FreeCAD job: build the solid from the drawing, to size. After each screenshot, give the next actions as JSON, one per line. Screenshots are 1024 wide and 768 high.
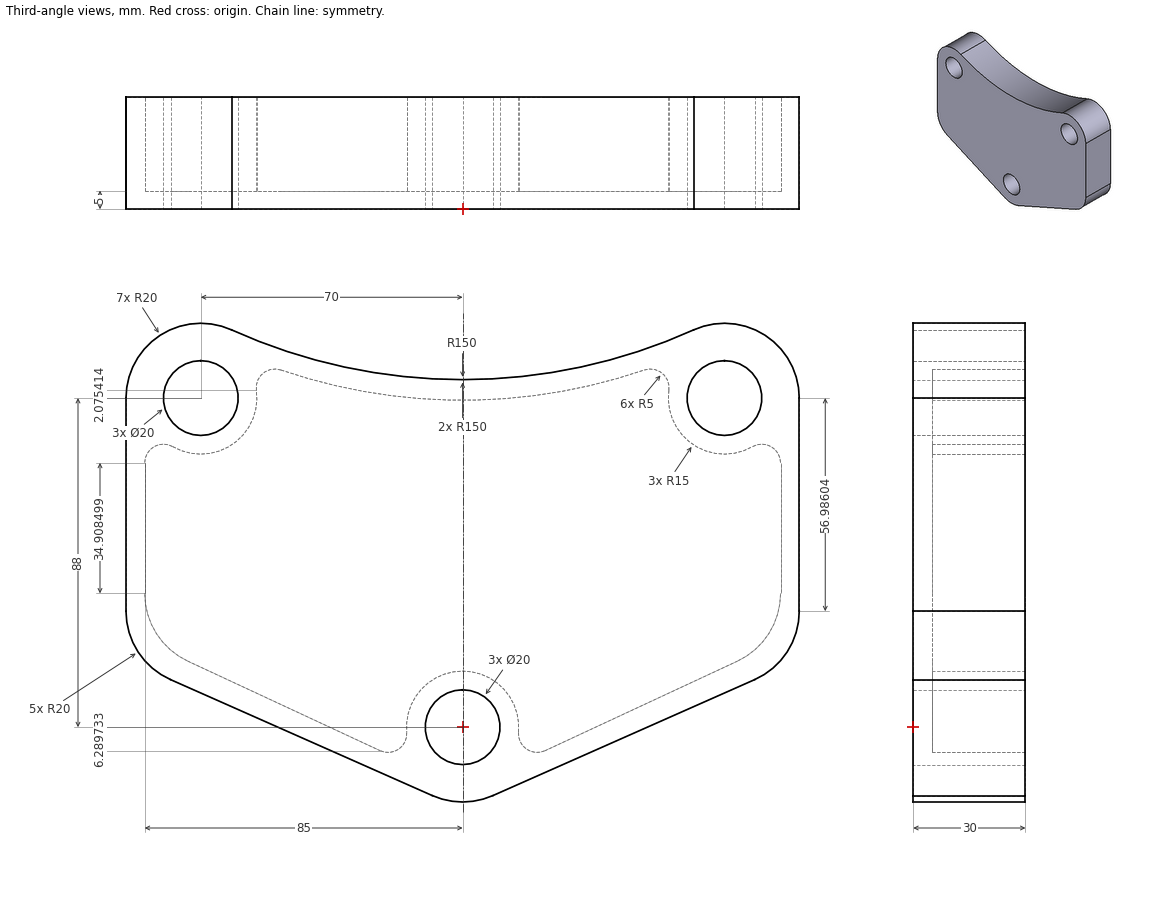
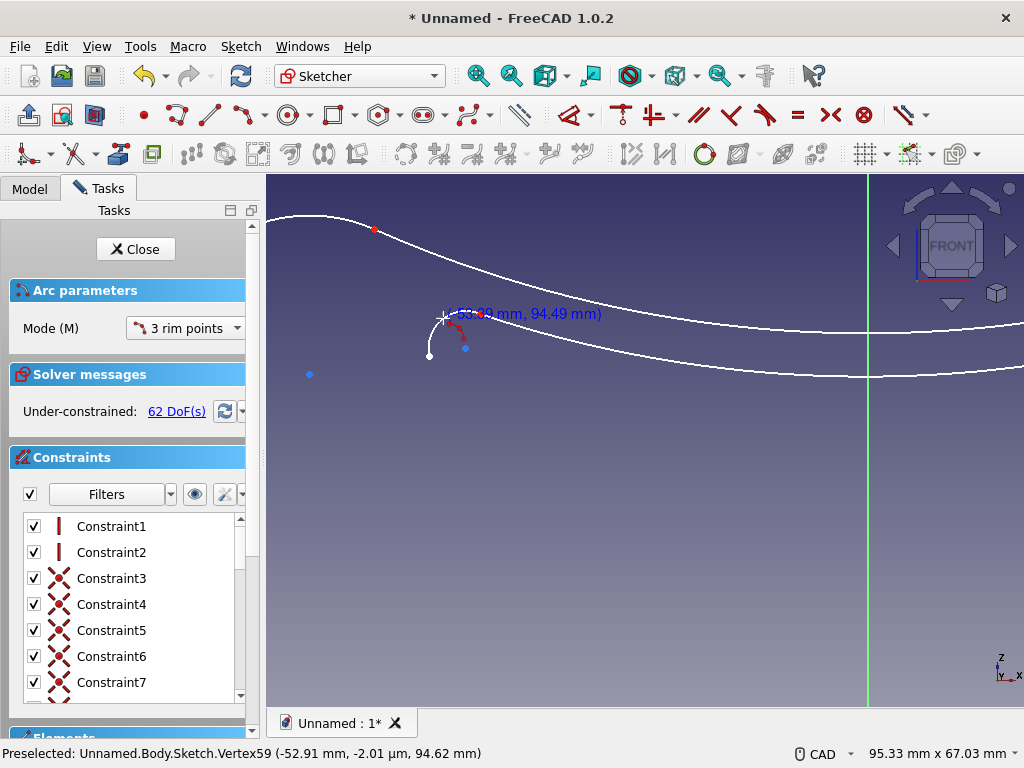
{"action": "left_click", "coordinate": [429, 357]}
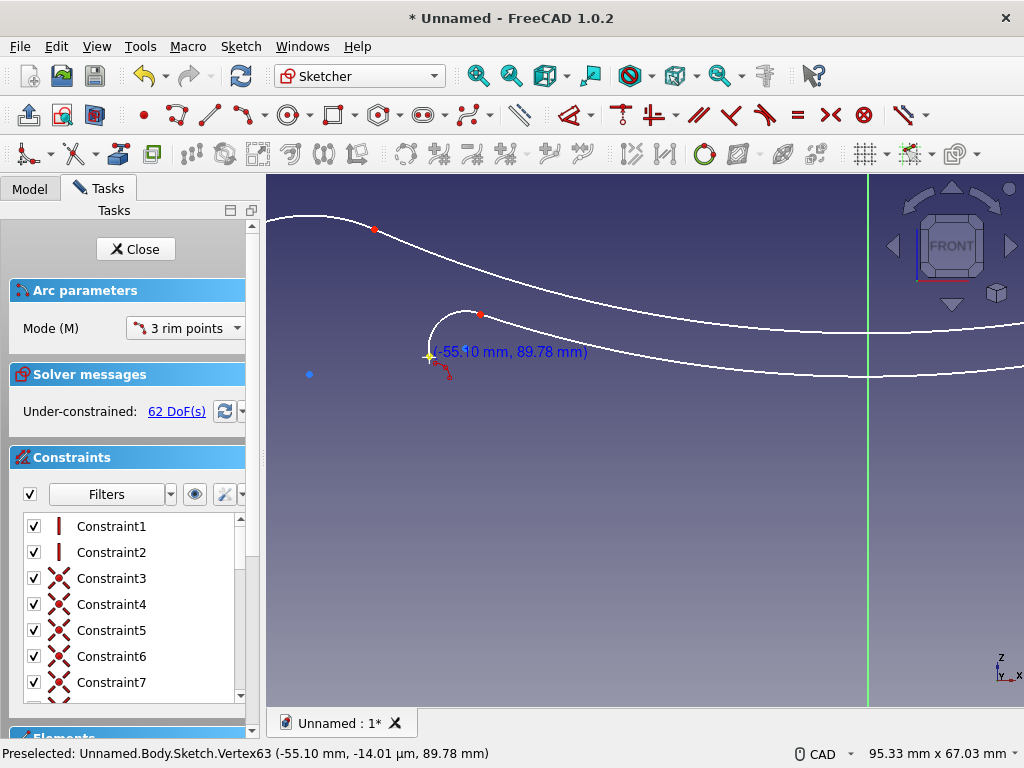
{"action": "scroll", "coordinate": [451, 317], "scroll_direction": "down", "scroll_amount": 6}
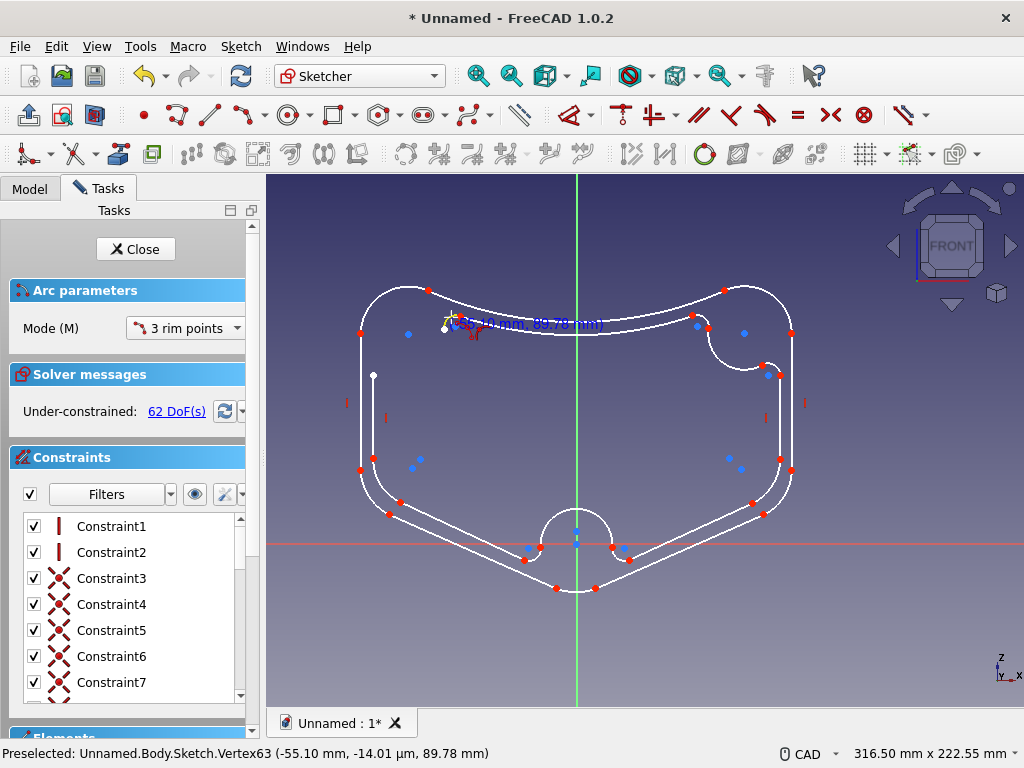
{"action": "left_click", "coordinate": [391, 364]}
{"action": "left_click", "coordinate": [429, 363]}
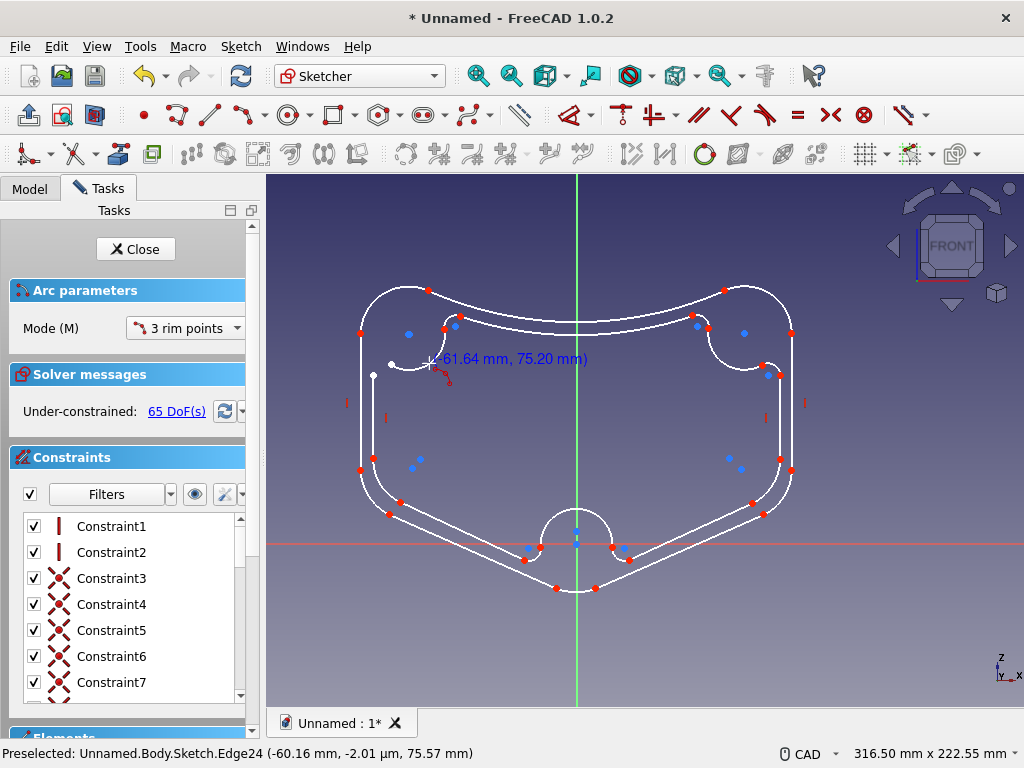
{"action": "left_click", "coordinate": [391, 365]}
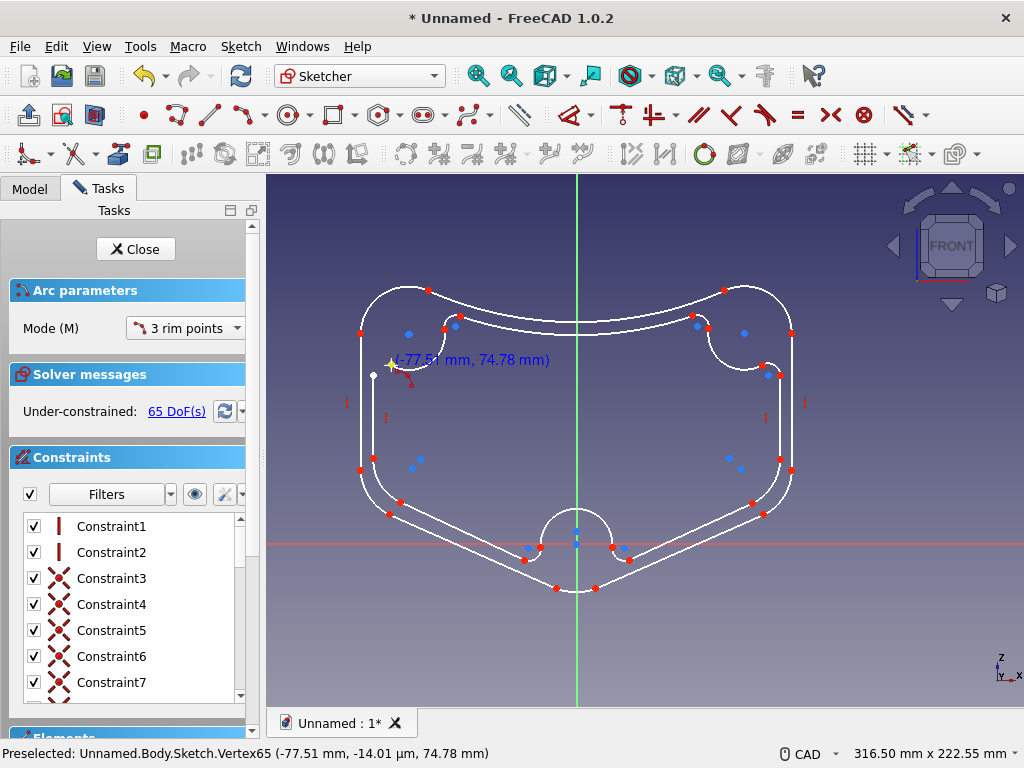
{"action": "scroll", "coordinate": [373, 375], "scroll_direction": "up", "scroll_amount": 2}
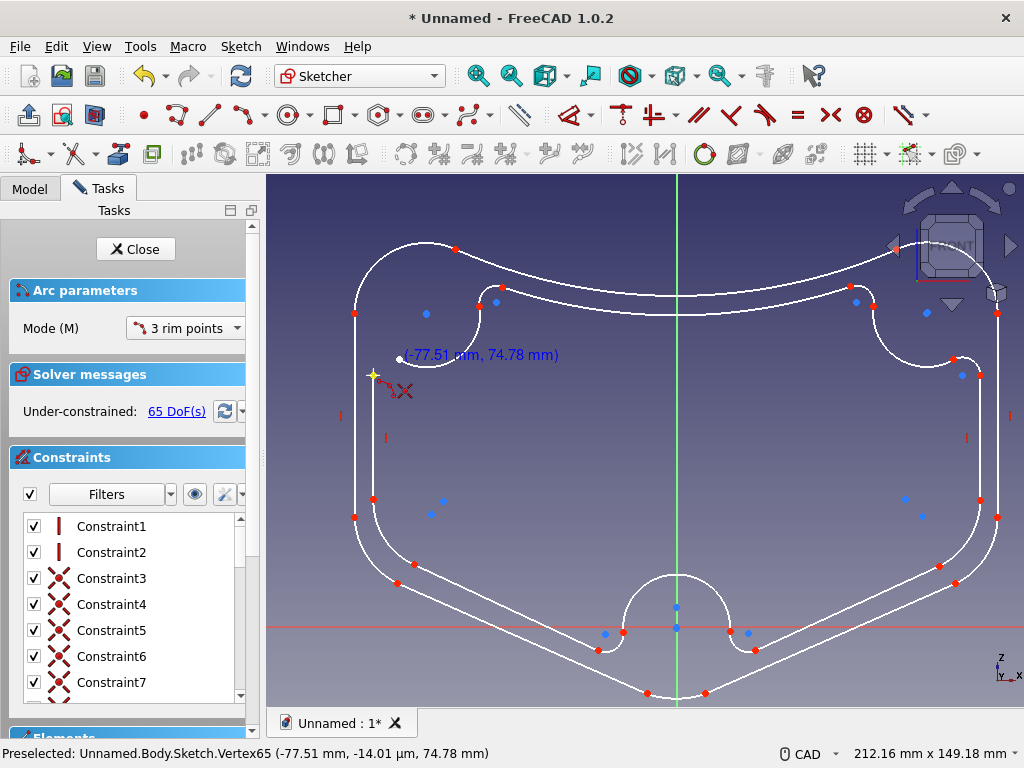
{"action": "left_click", "coordinate": [373, 376]}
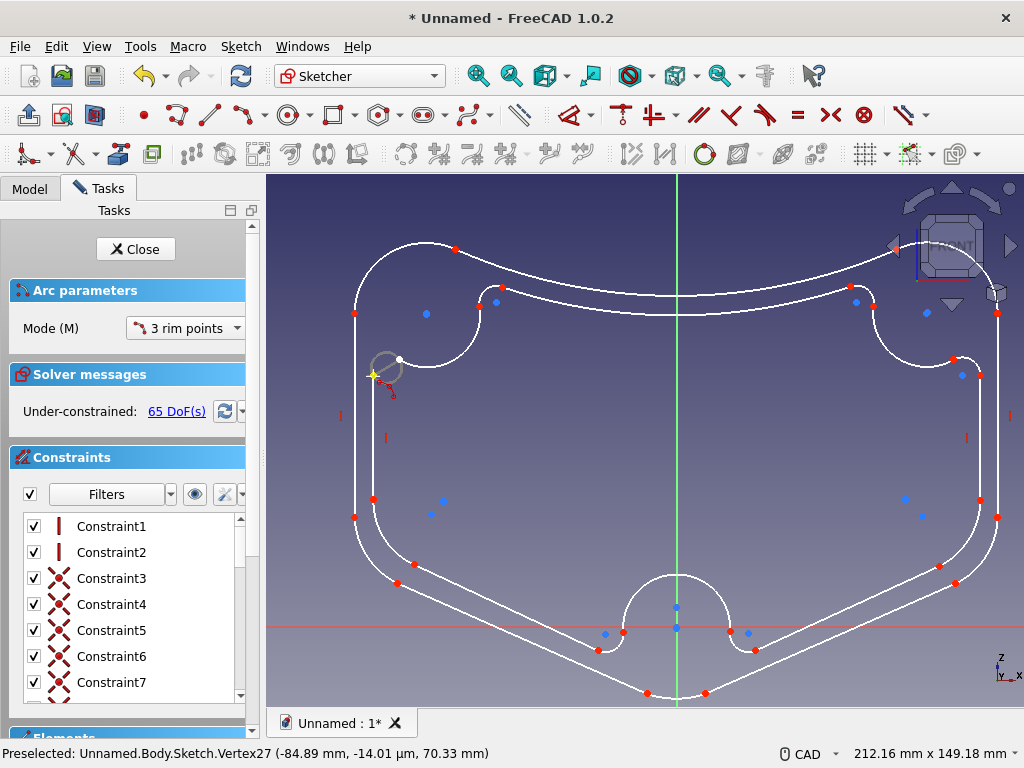
{"action": "scroll", "coordinate": [382, 359], "scroll_direction": "up", "scroll_amount": 3}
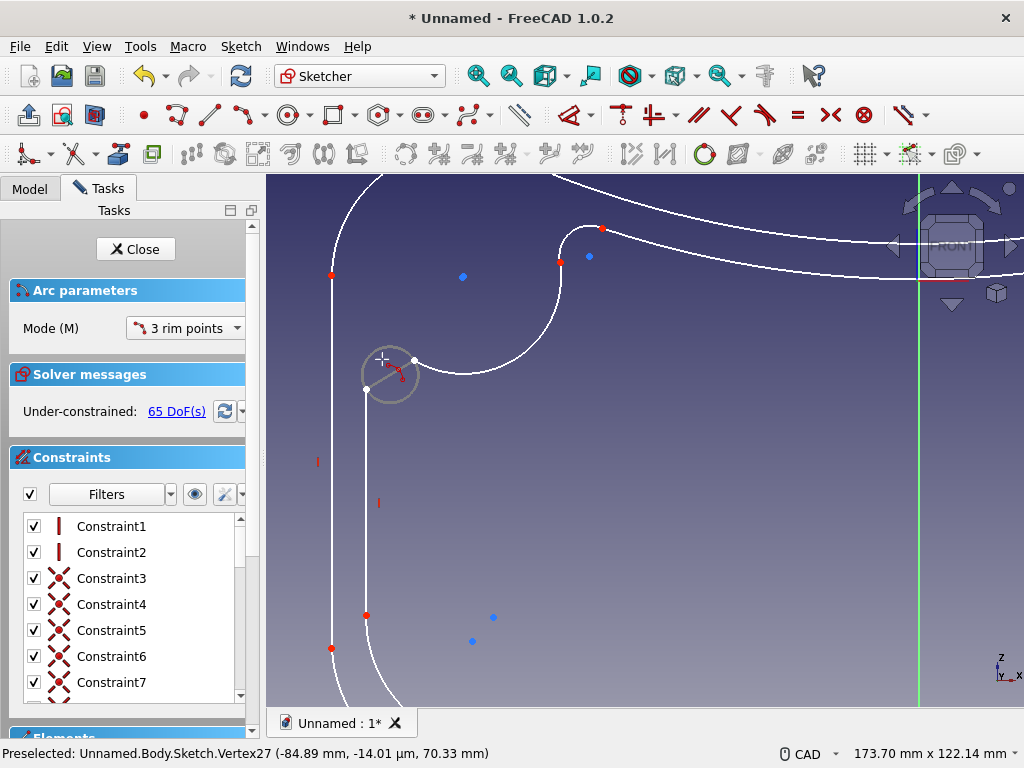
{"action": "left_click", "coordinate": [382, 359]}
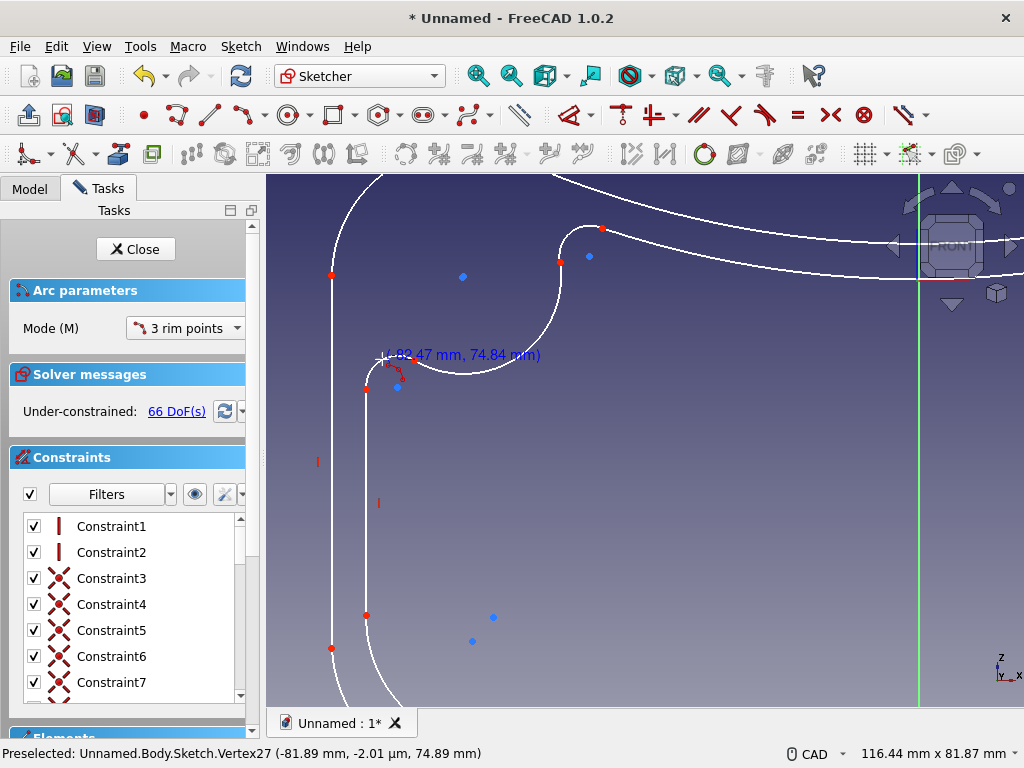
{"action": "left_click", "coordinate": [288, 116]}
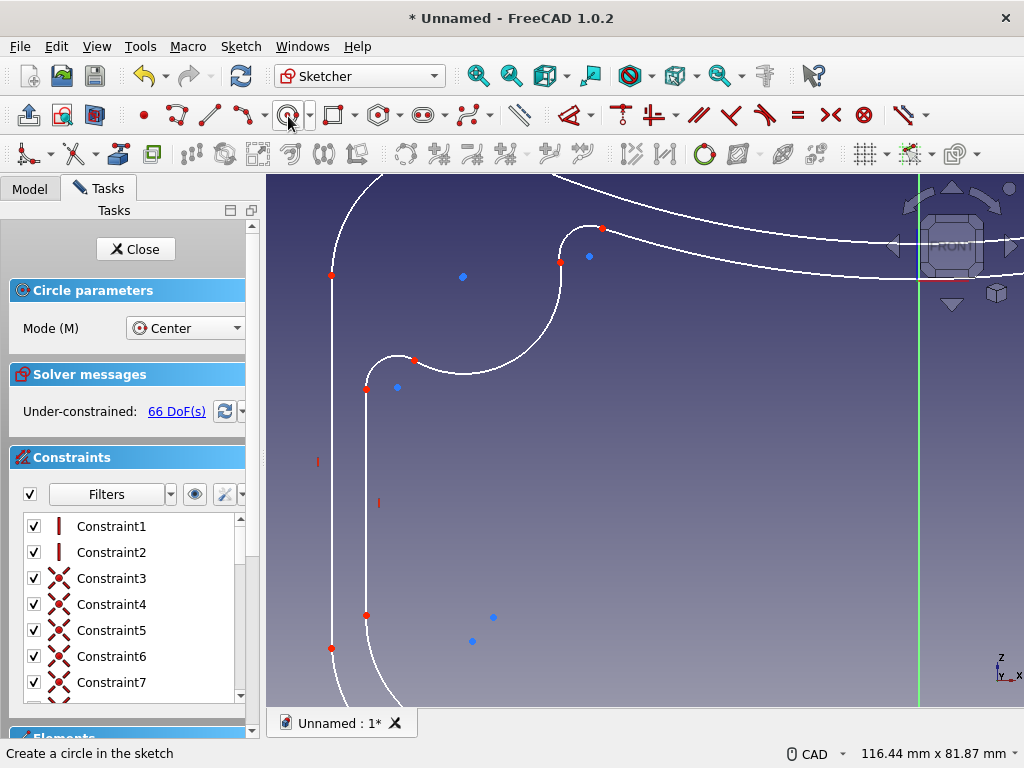
{"action": "left_click", "coordinate": [463, 274]}
{"action": "left_click", "coordinate": [509, 228]}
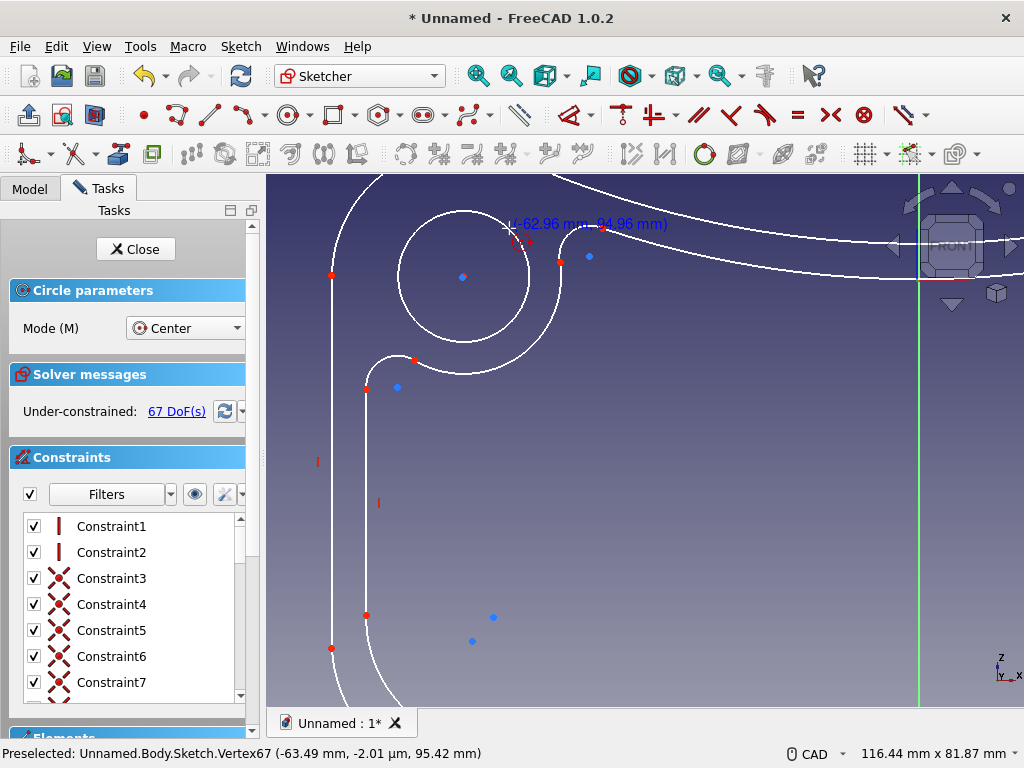
{"action": "scroll", "coordinate": [377, 367], "scroll_direction": "down", "scroll_amount": 5}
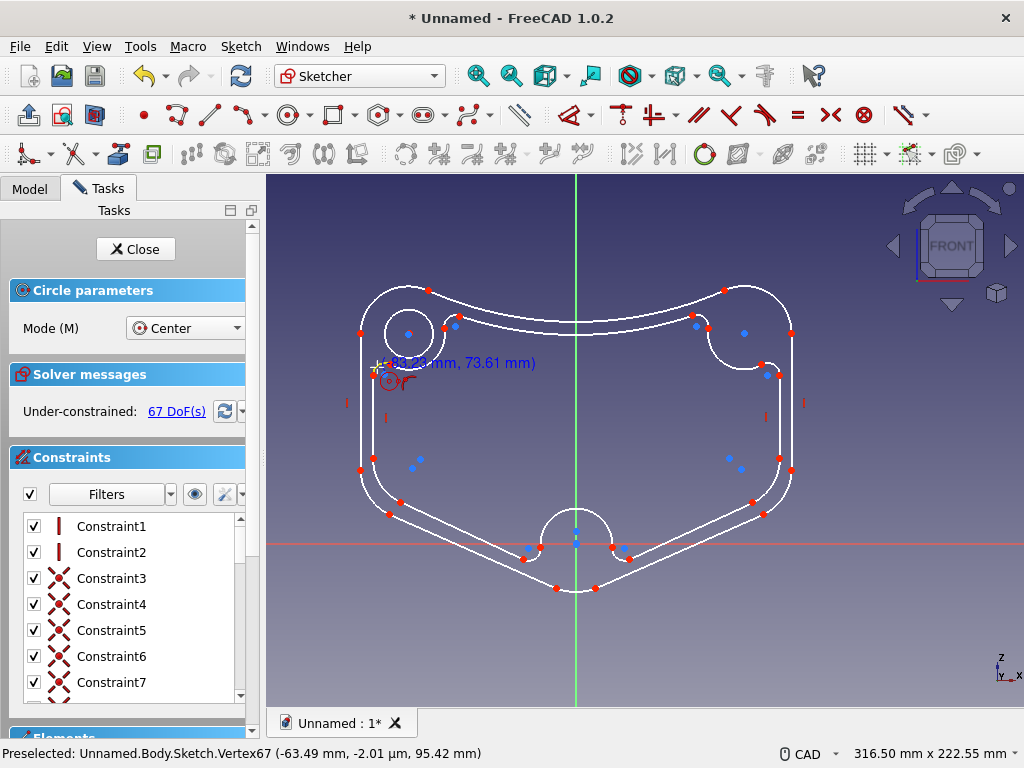
{"action": "left_click", "coordinate": [744, 333]}
{"action": "left_click", "coordinate": [761, 316]}